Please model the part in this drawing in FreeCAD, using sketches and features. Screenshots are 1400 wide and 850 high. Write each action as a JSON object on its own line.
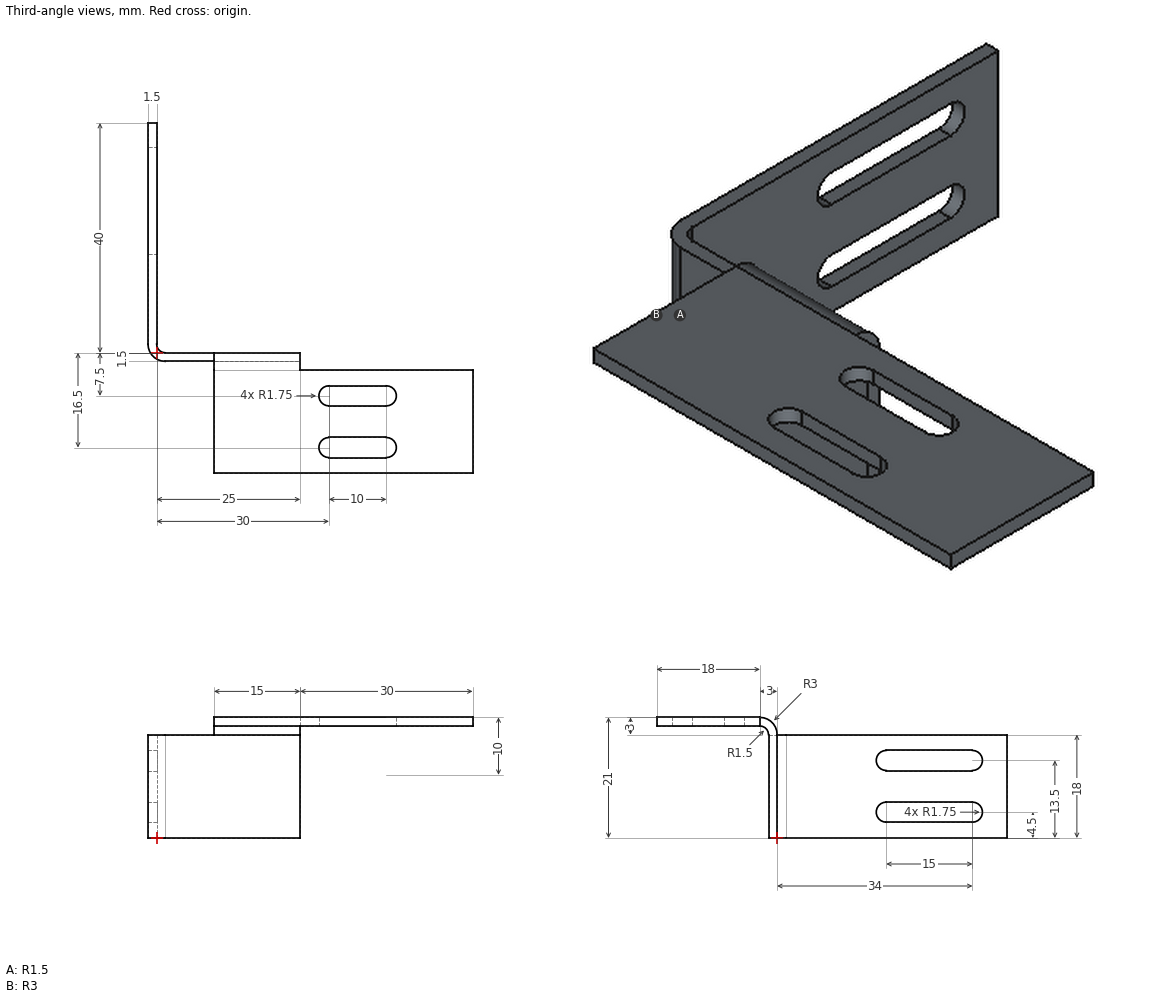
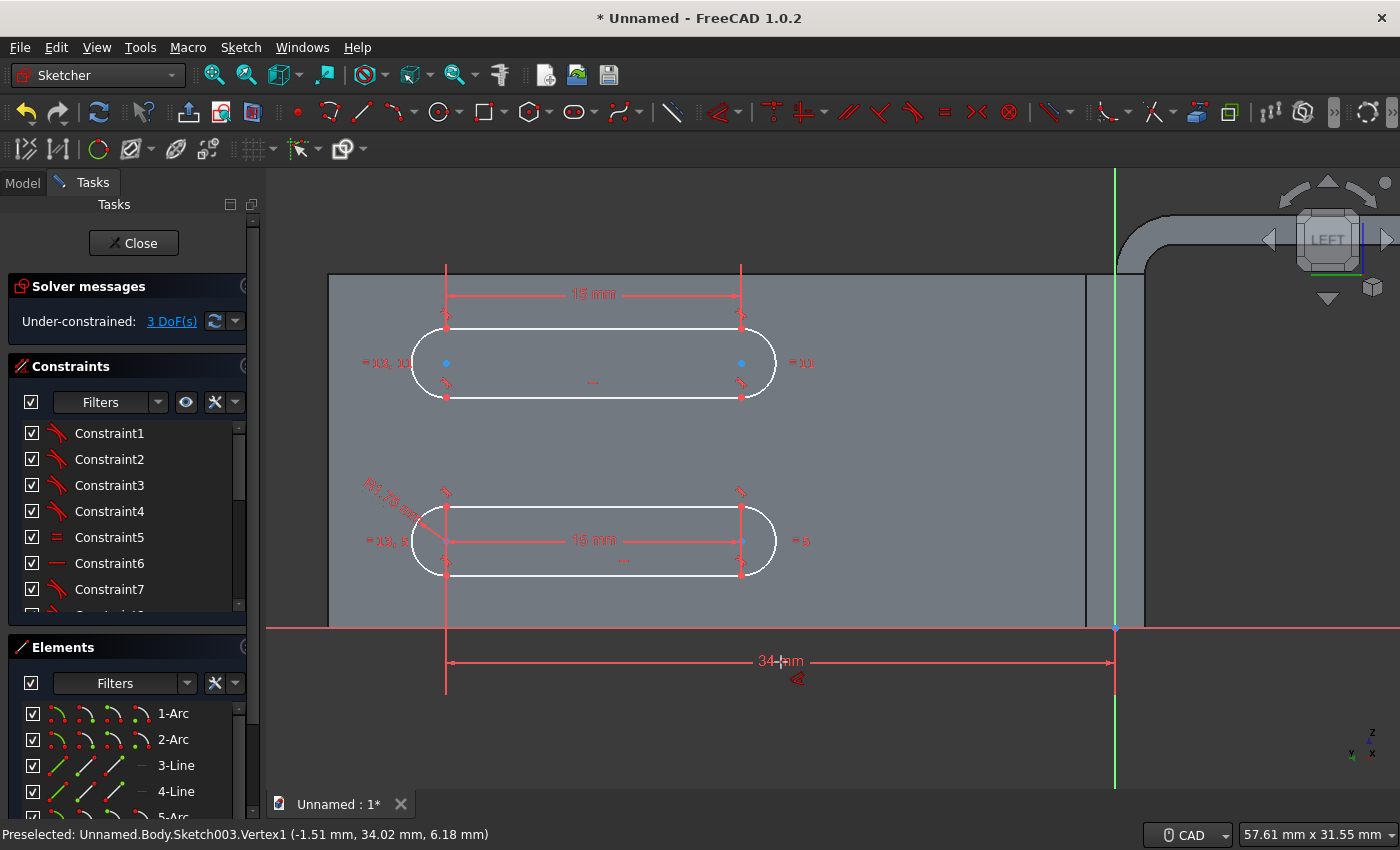
{"action": "left_click", "coordinate": [446, 329]}
{"action": "left_click", "coordinate": [627, 662]}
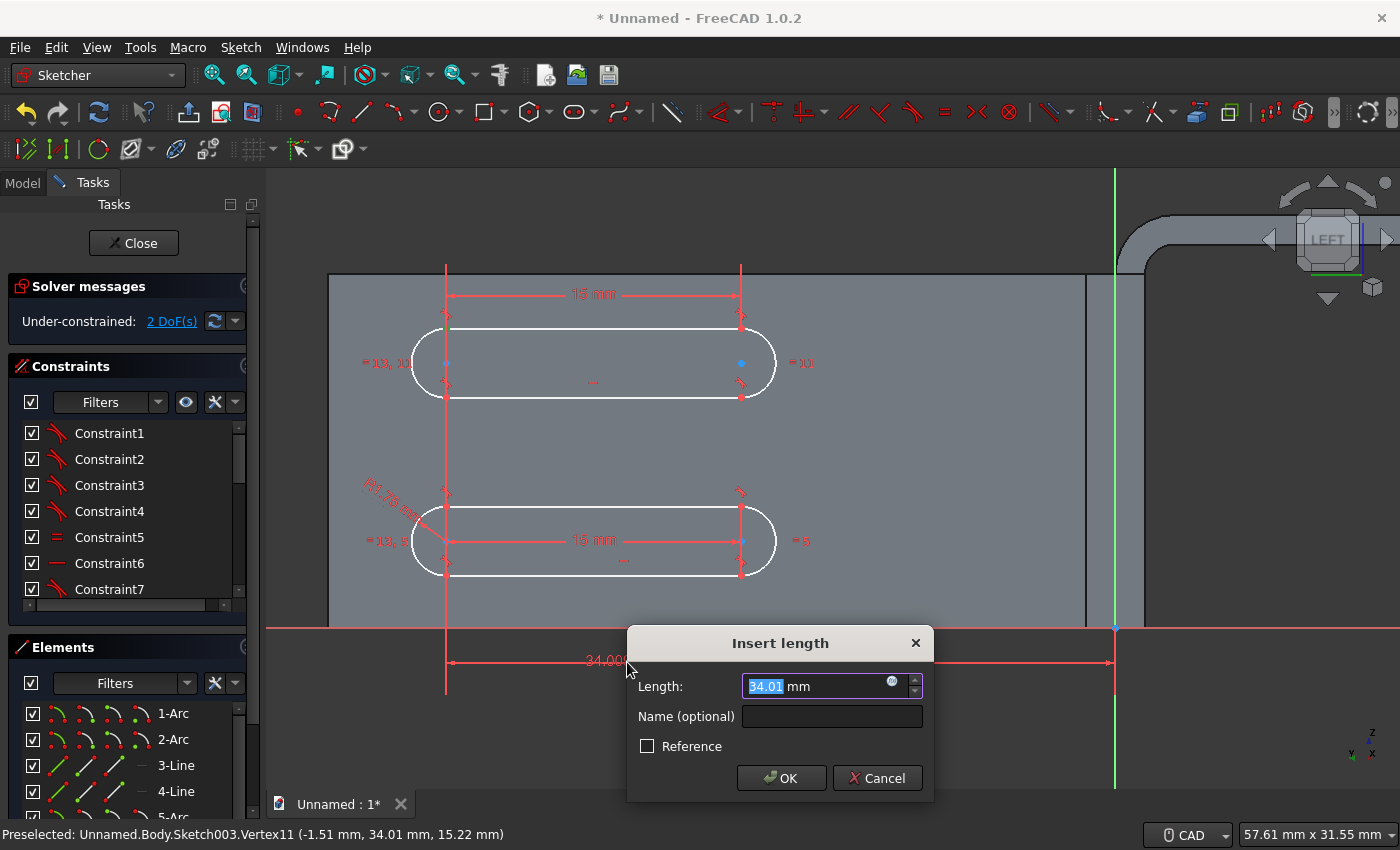
{"action": "type", "text": "34"}
{"action": "key", "text": "Return"}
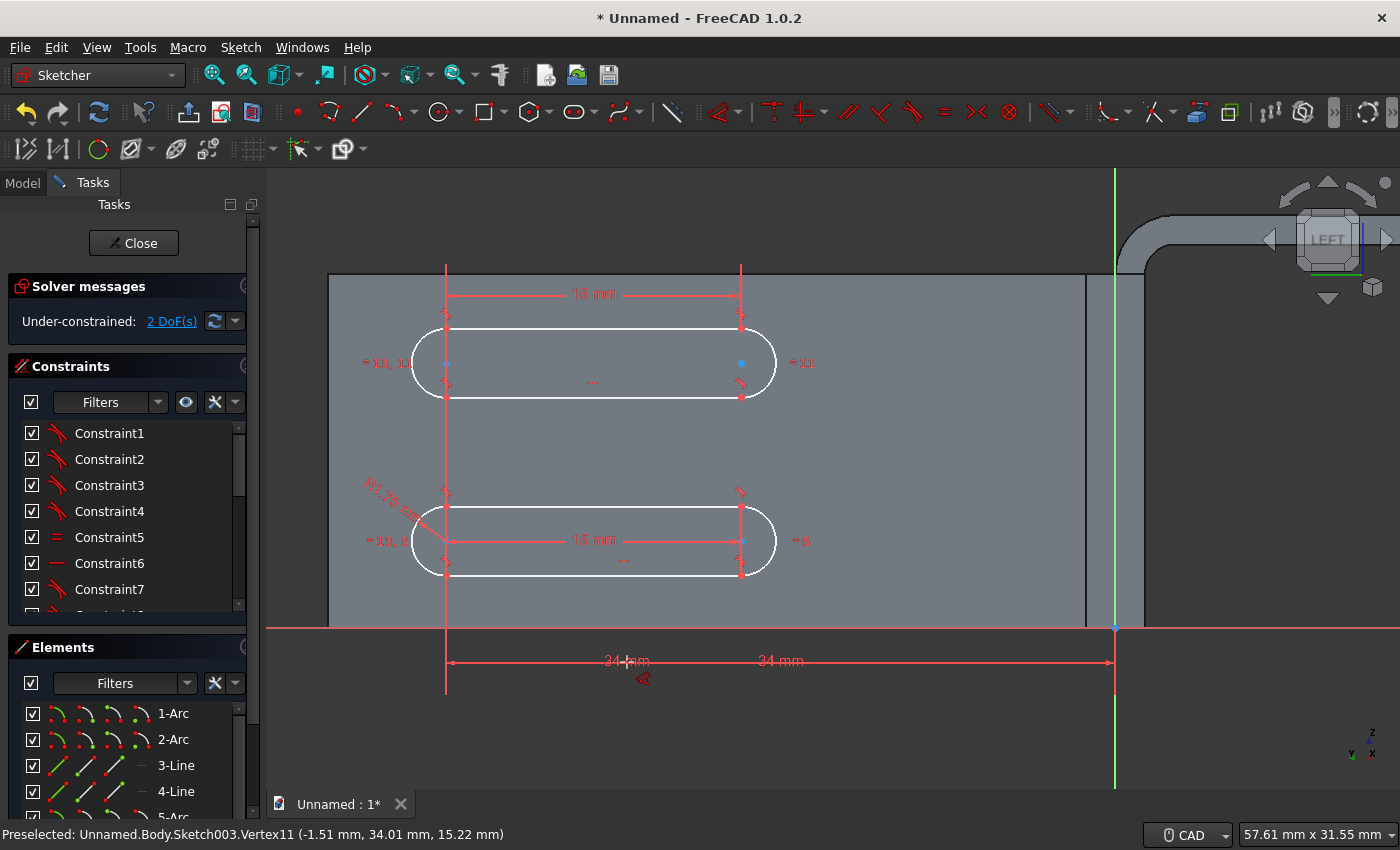
{"action": "left_click", "coordinate": [446, 541]}
{"action": "left_click", "coordinate": [1149, 585]}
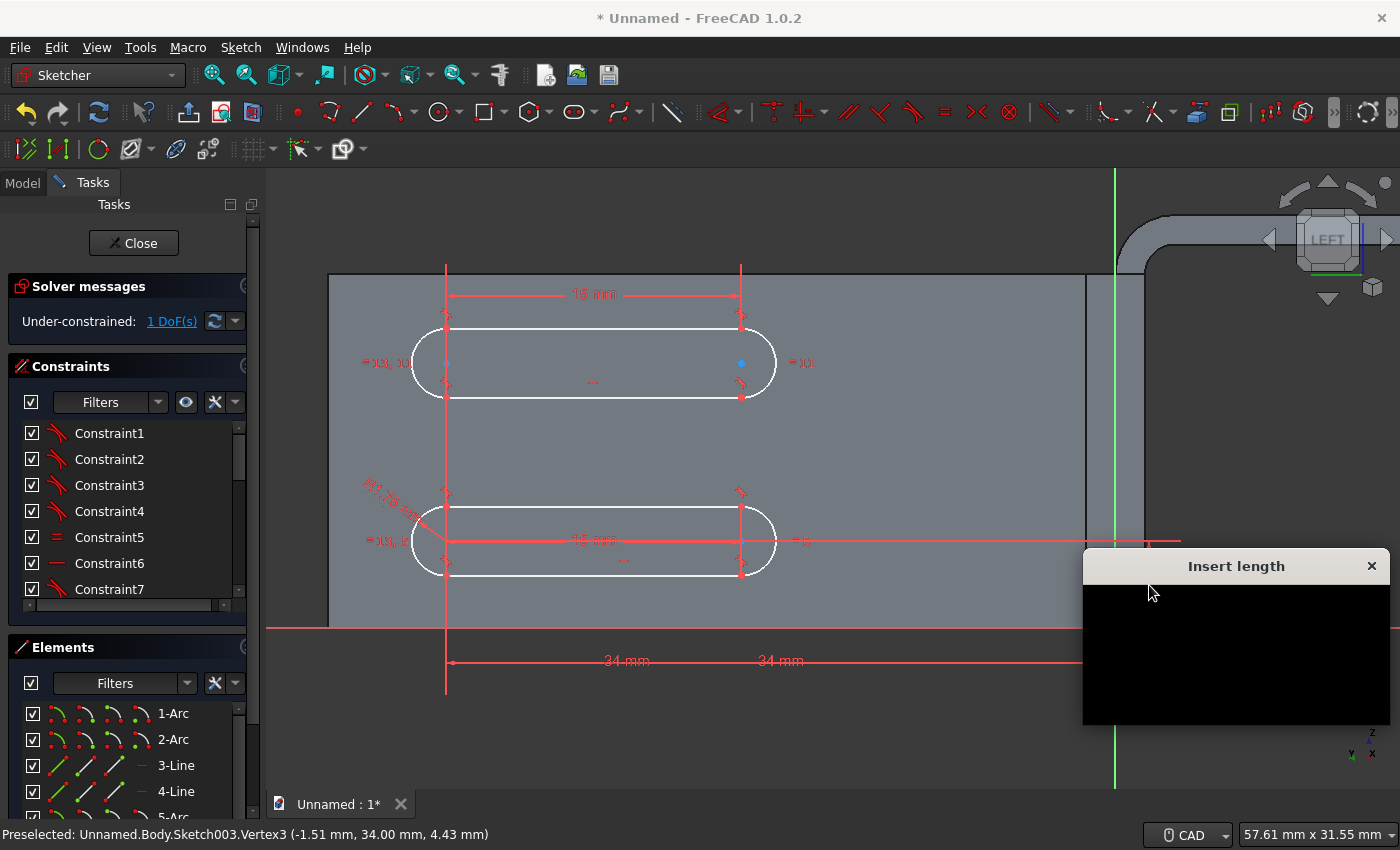
{"action": "type", "text": "4.5"}
{"action": "key", "text": "Return"}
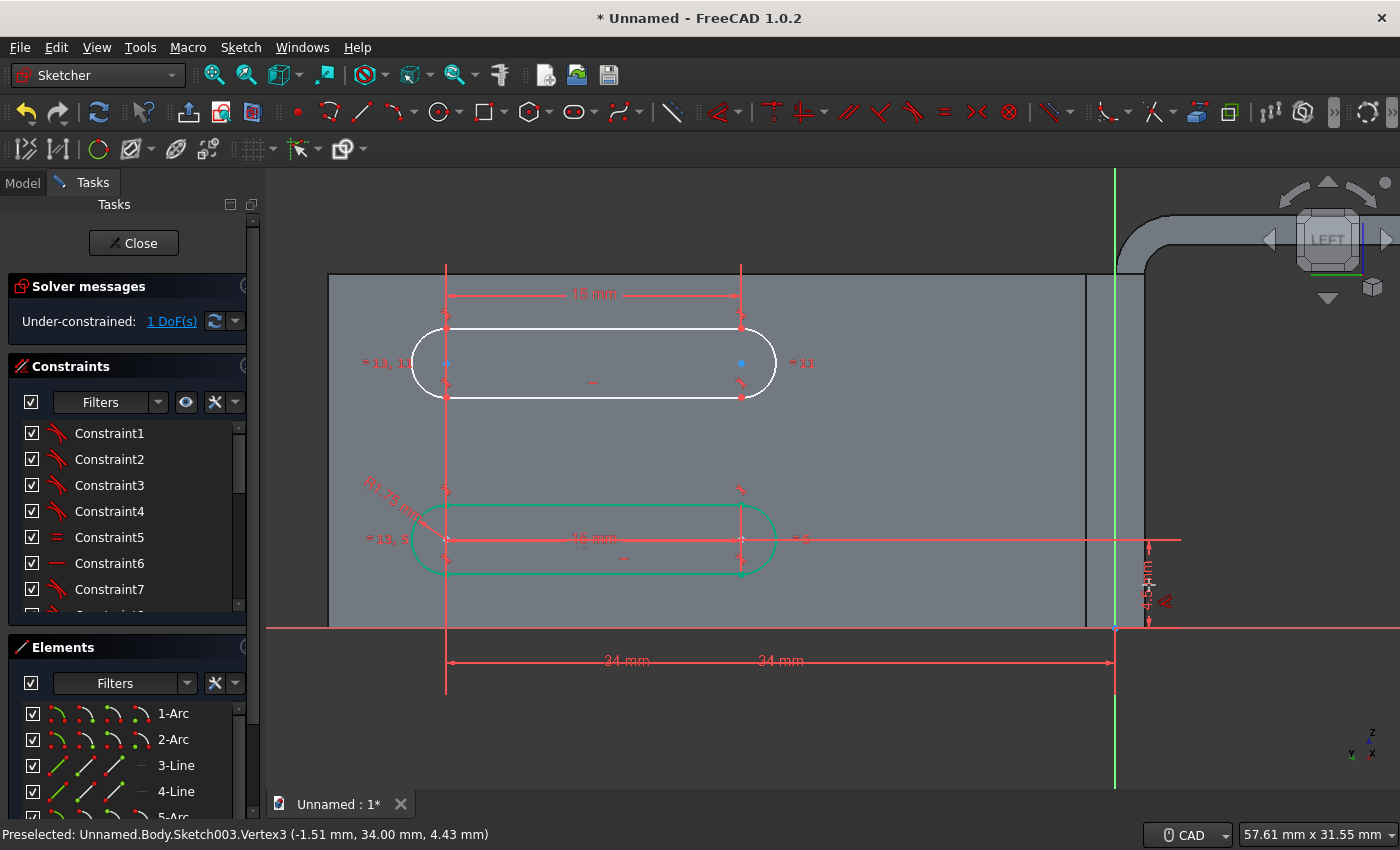
{"action": "left_click", "coordinate": [446, 363]}
{"action": "left_click", "coordinate": [1149, 496]}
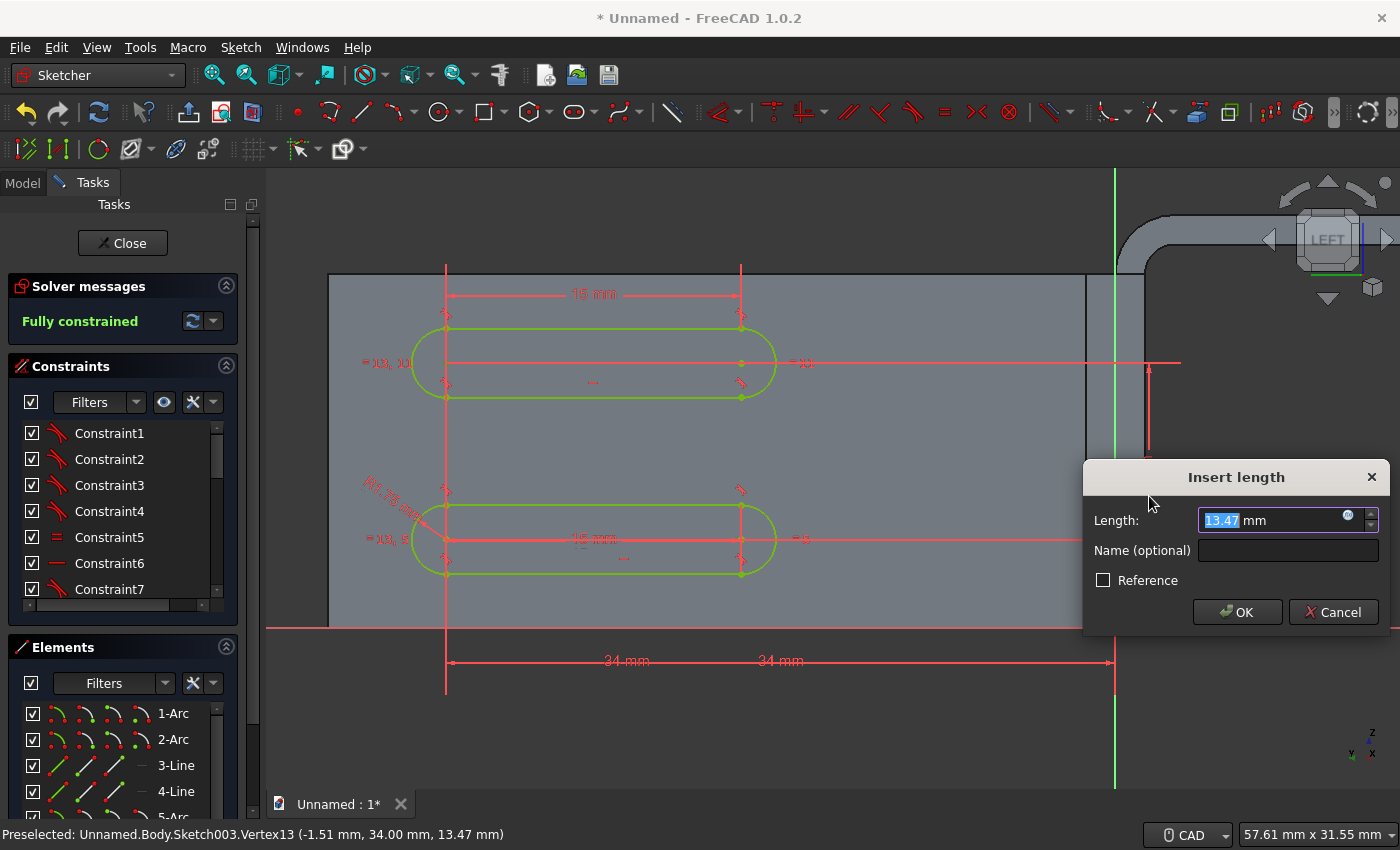
{"action": "type", "text": "13.5"}
{"action": "key", "text": "Return"}
{"action": "key", "text": "Escape"}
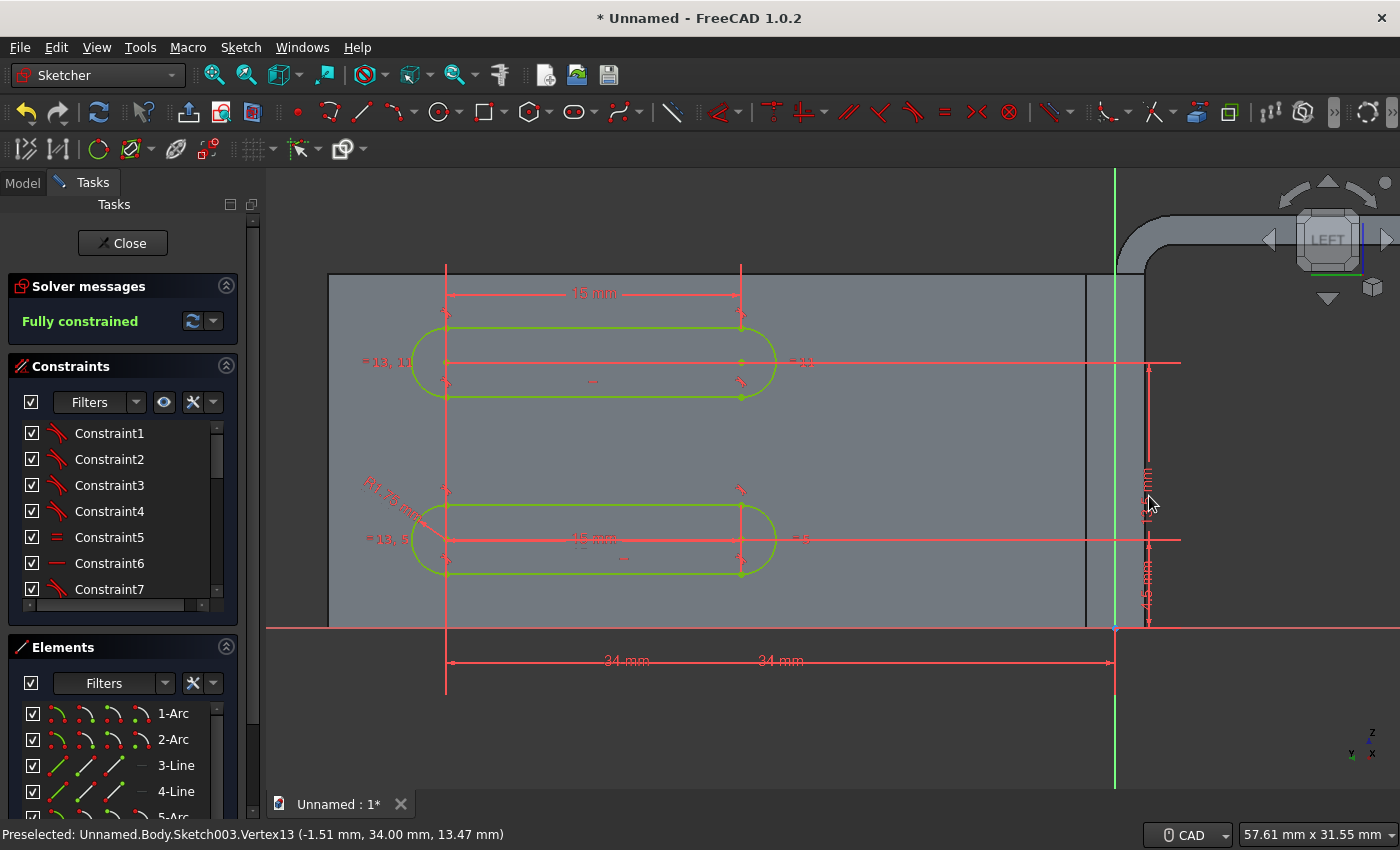
{"action": "left_click", "coordinate": [123, 243]}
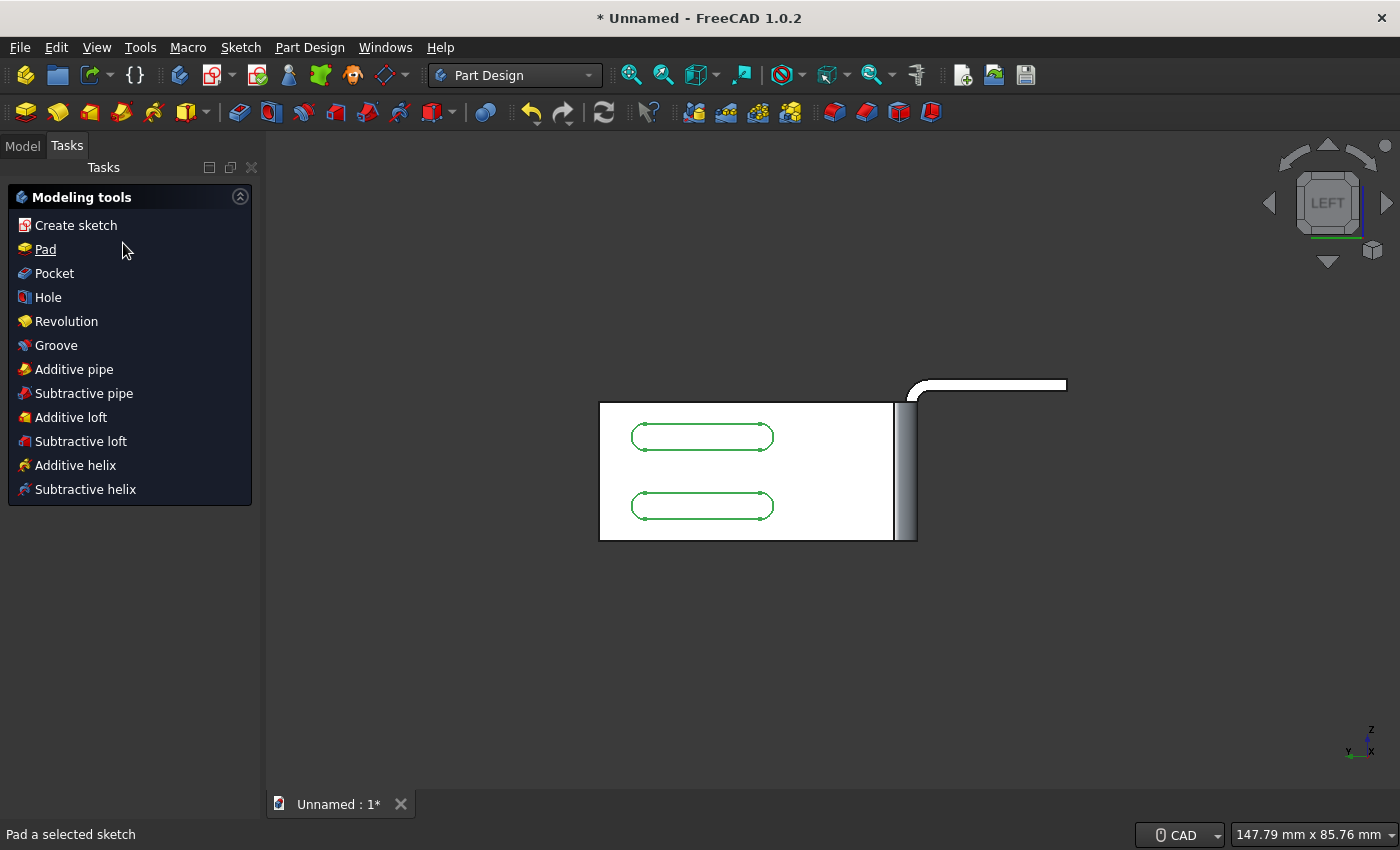
{"action": "left_click", "coordinate": [240, 112]}